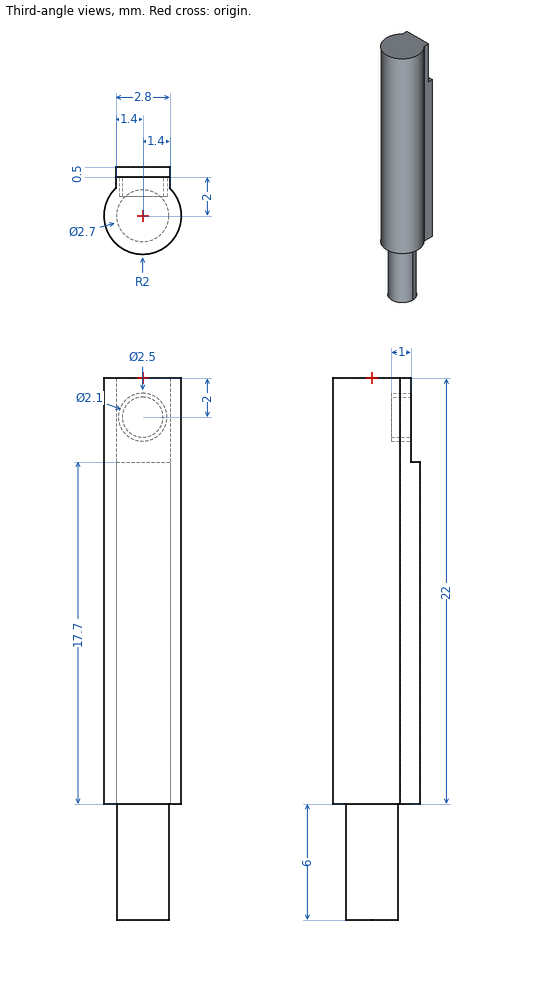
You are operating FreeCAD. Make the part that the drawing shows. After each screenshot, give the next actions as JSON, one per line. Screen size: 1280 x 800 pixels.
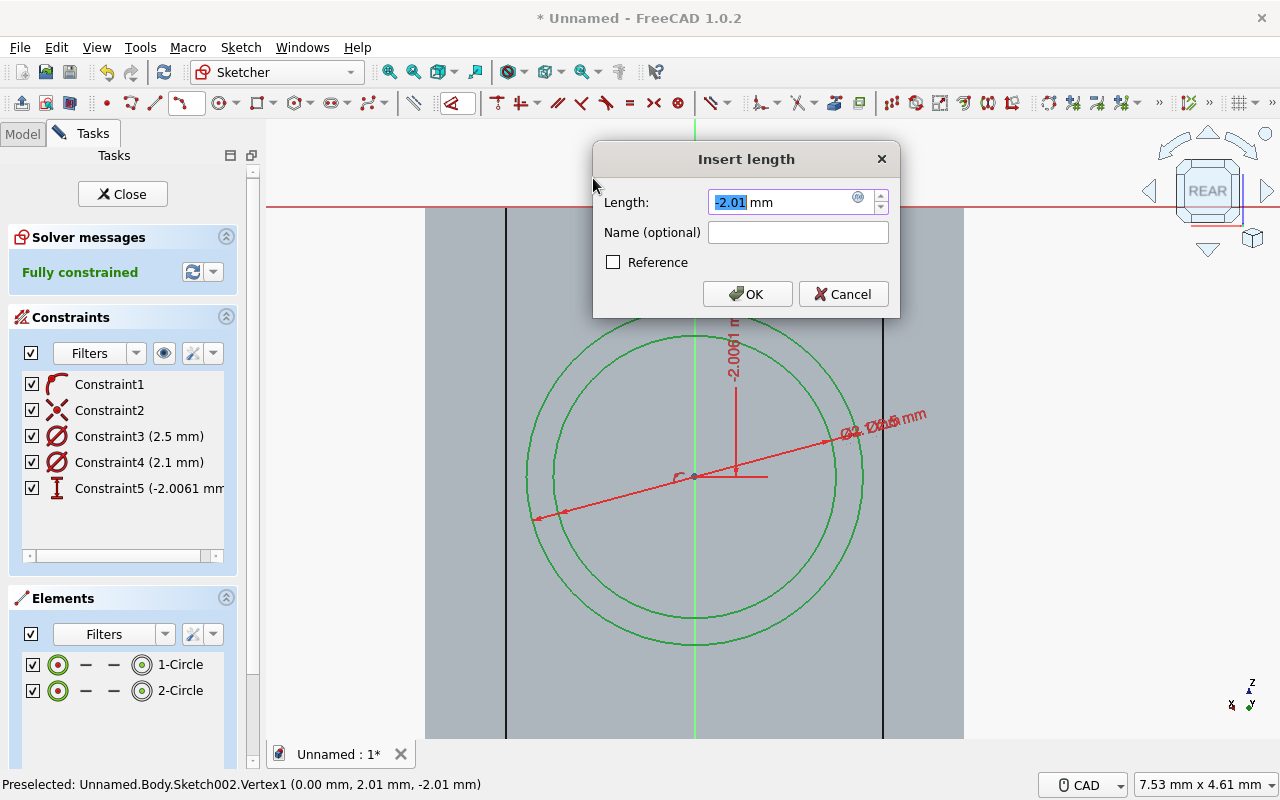
{"action": "type", "text": "-2"}
{"action": "key", "text": "Return"}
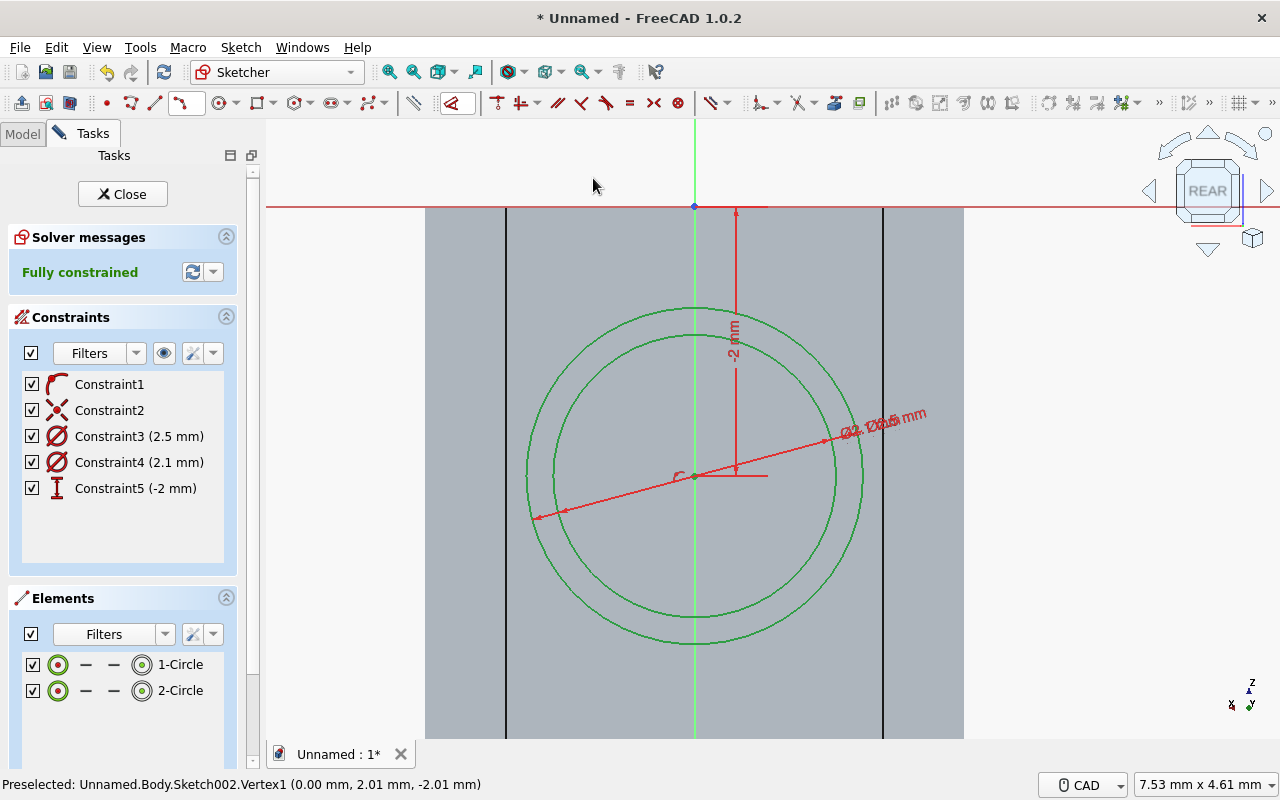
{"action": "left_click", "coordinate": [123, 194]}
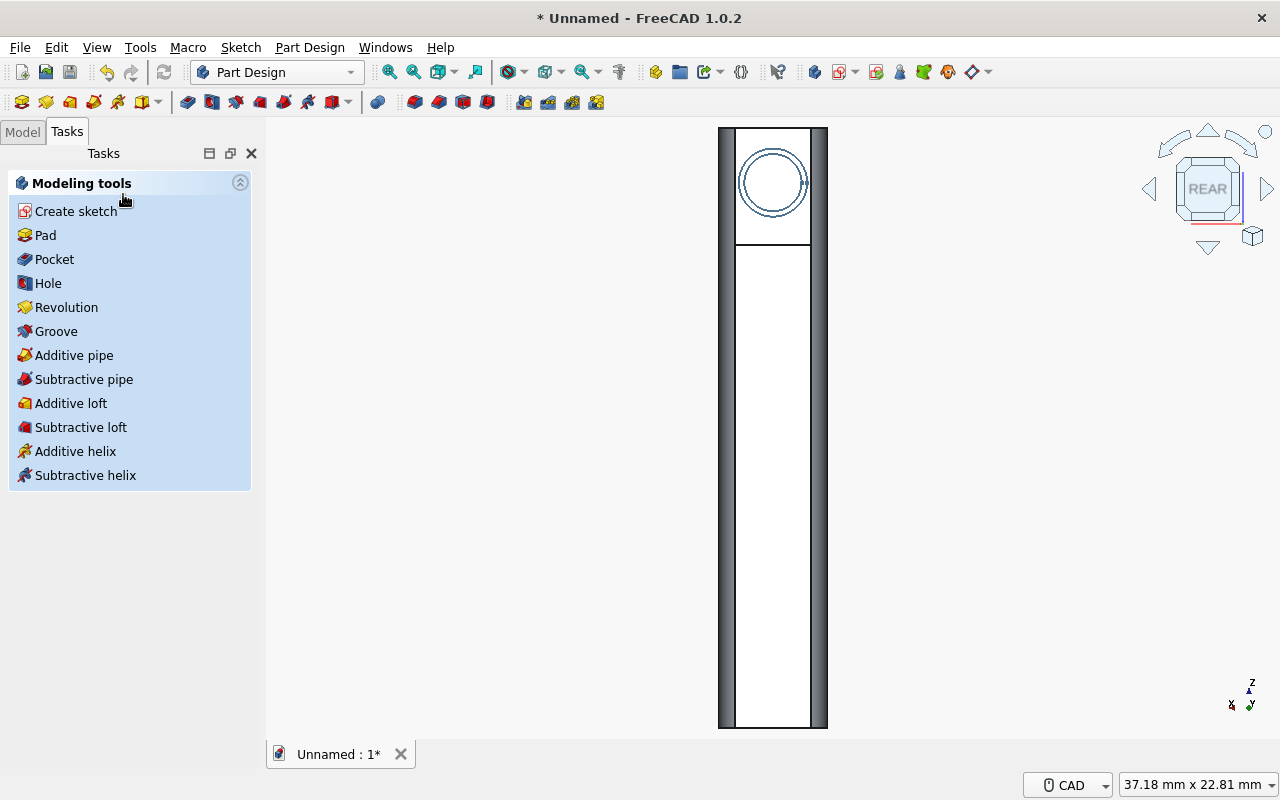
{"action": "left_click", "coordinate": [188, 102]}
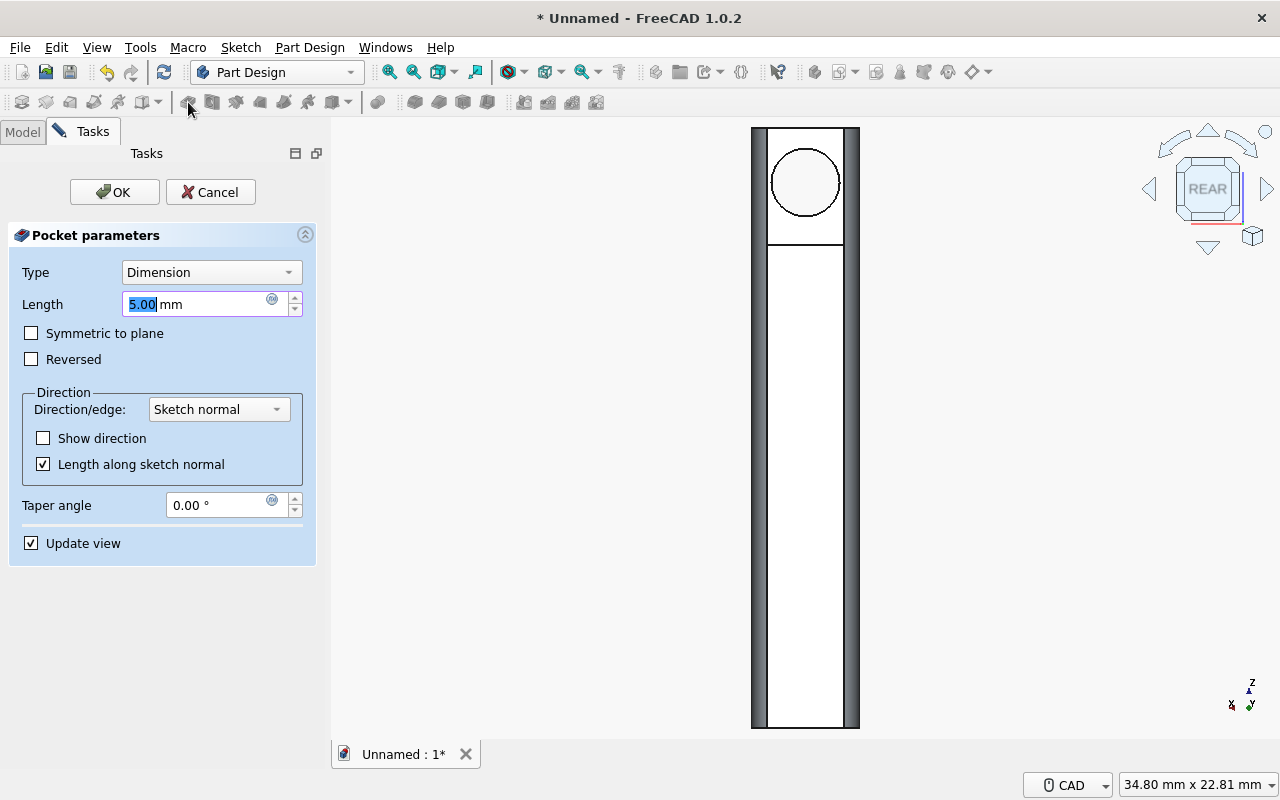
{"action": "type", "text": "1"}
{"action": "key", "text": "Tab"}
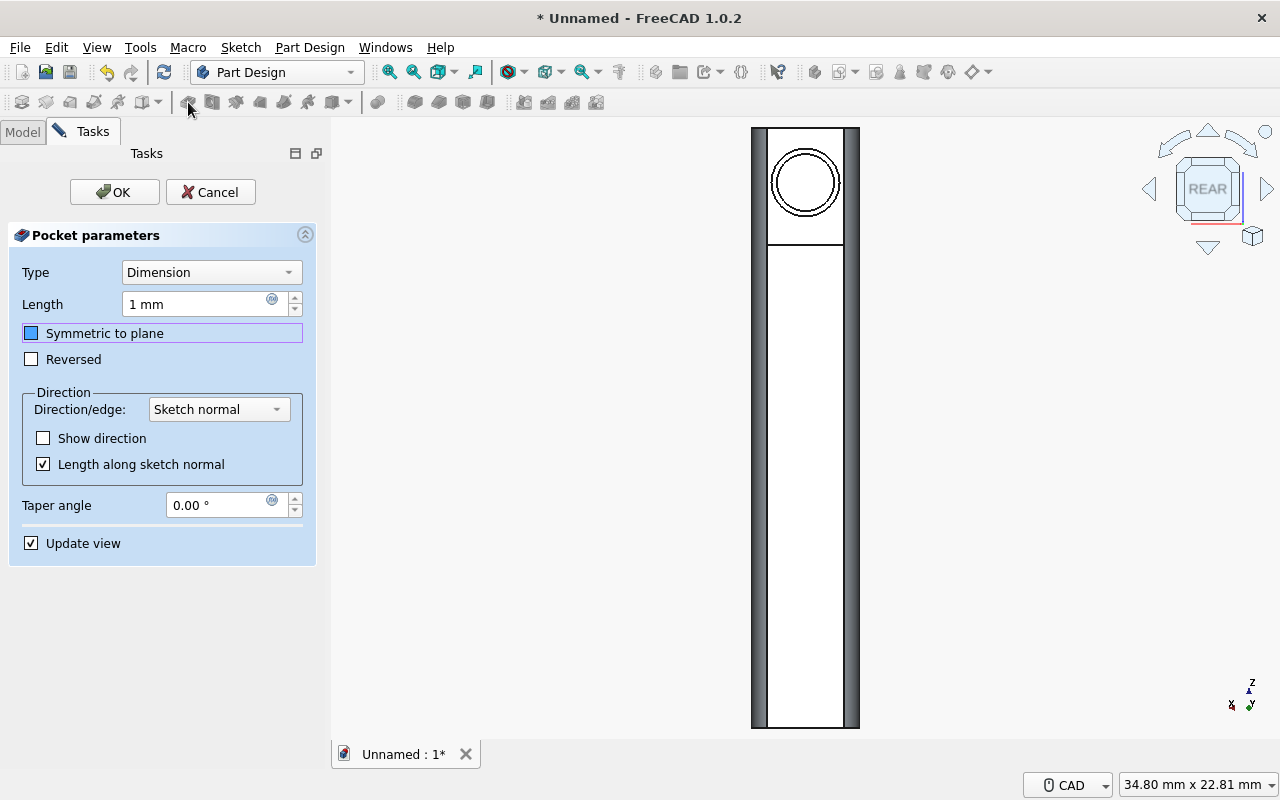
{"action": "left_click", "coordinate": [115, 192]}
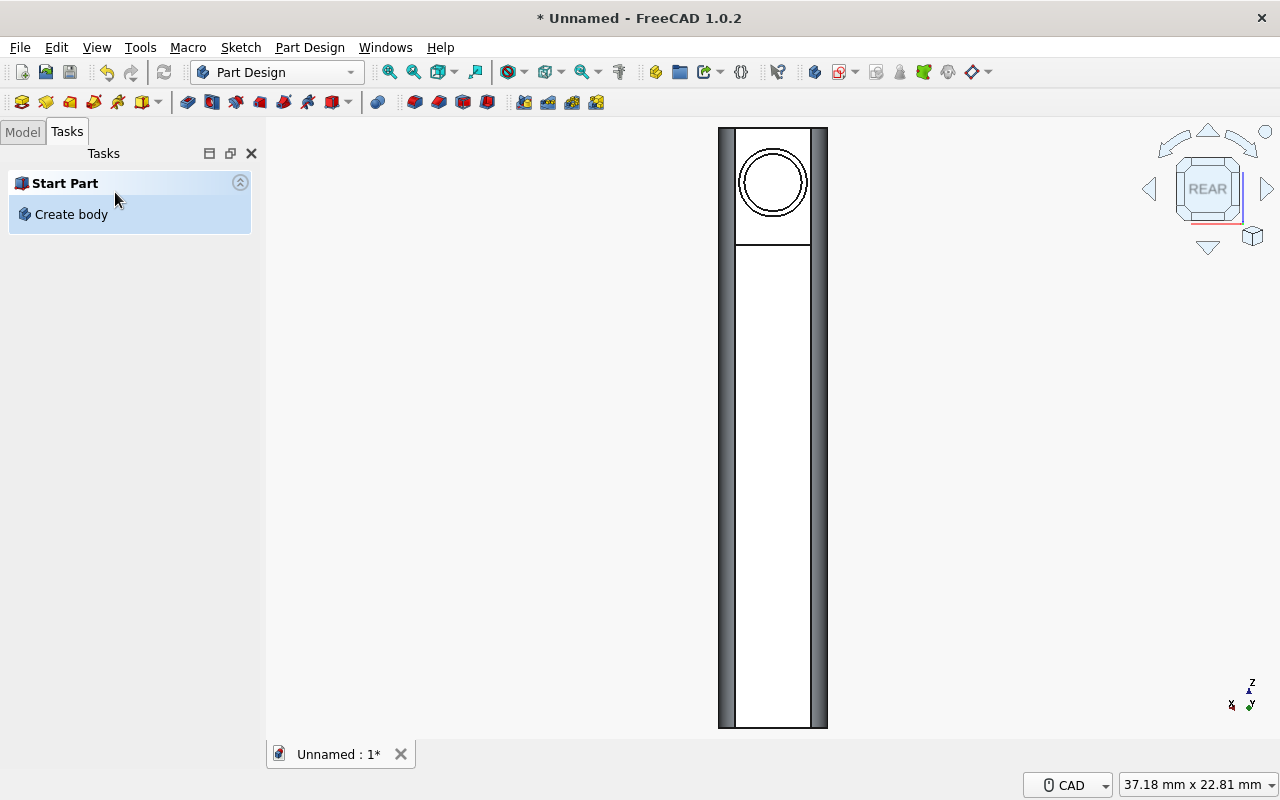
{"action": "key", "text": "5"}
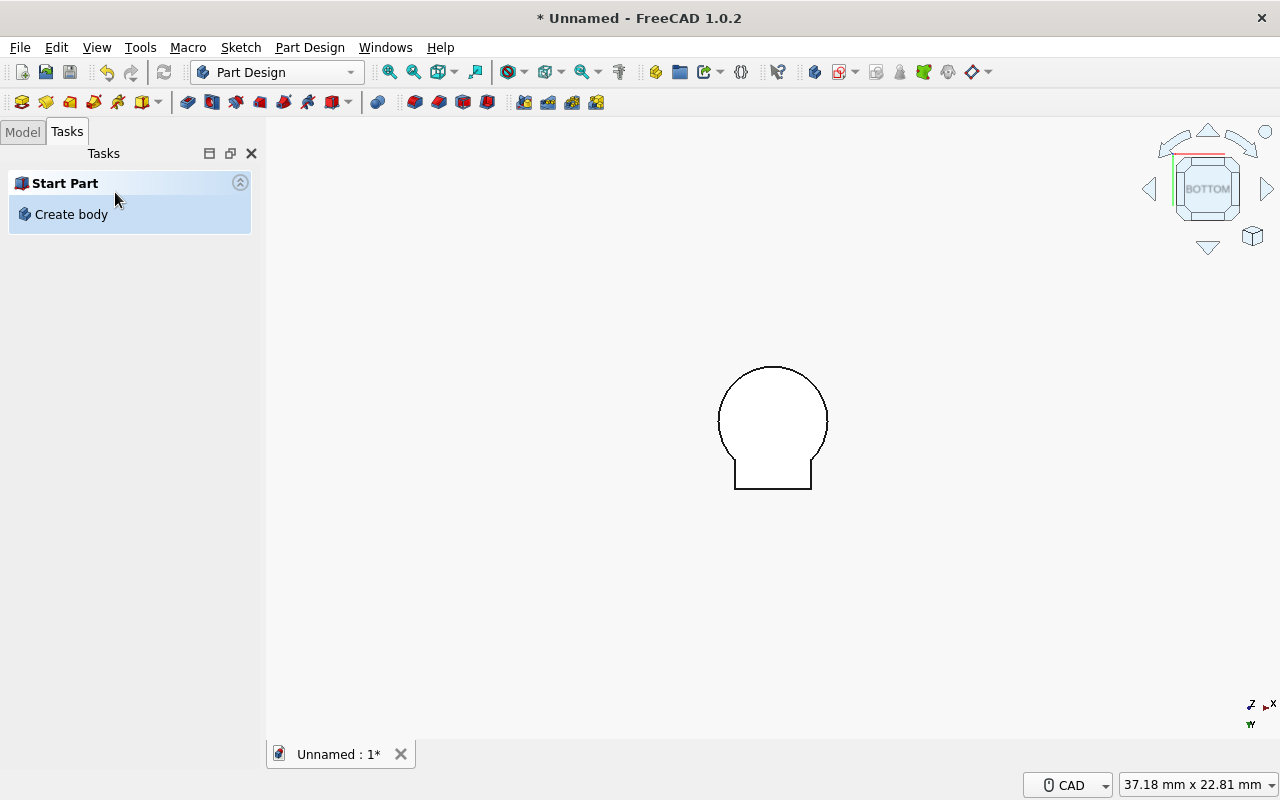
{"action": "left_click", "coordinate": [390, 72]}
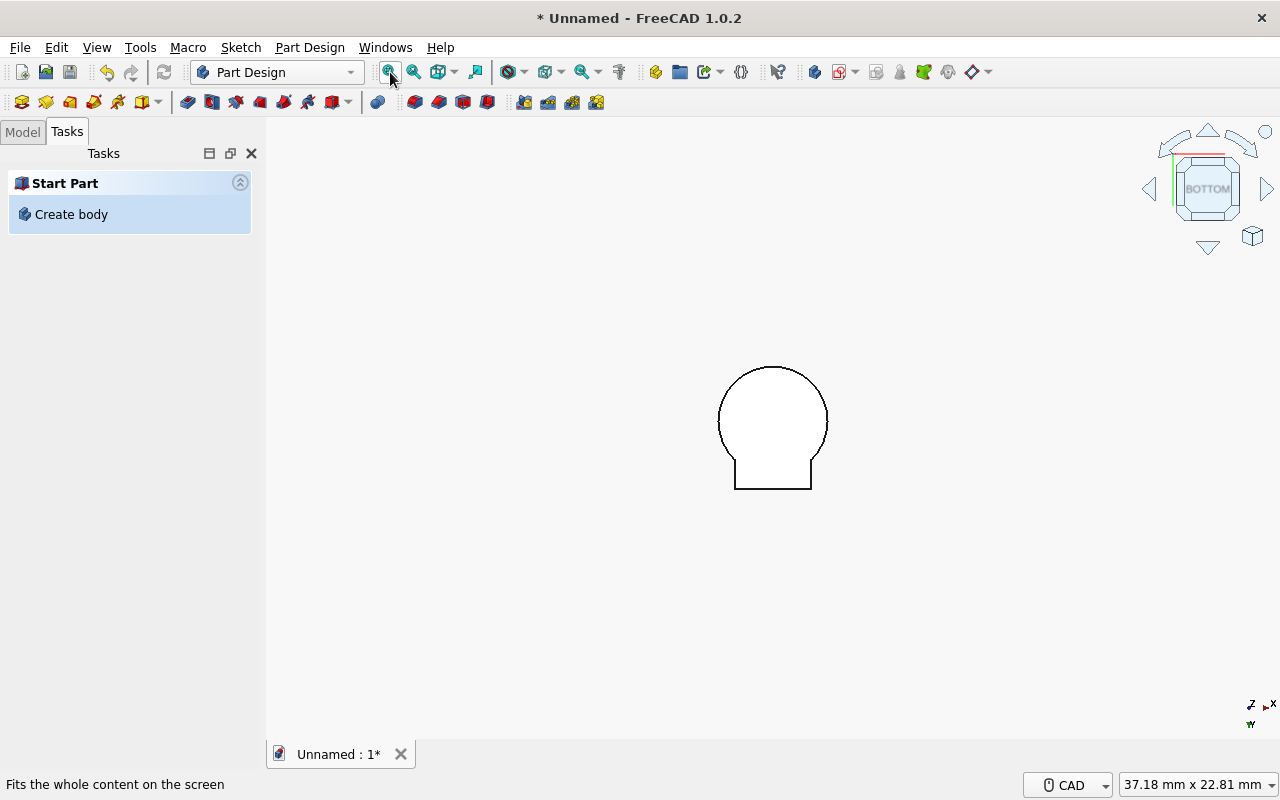
{"action": "left_click", "coordinate": [773, 427]}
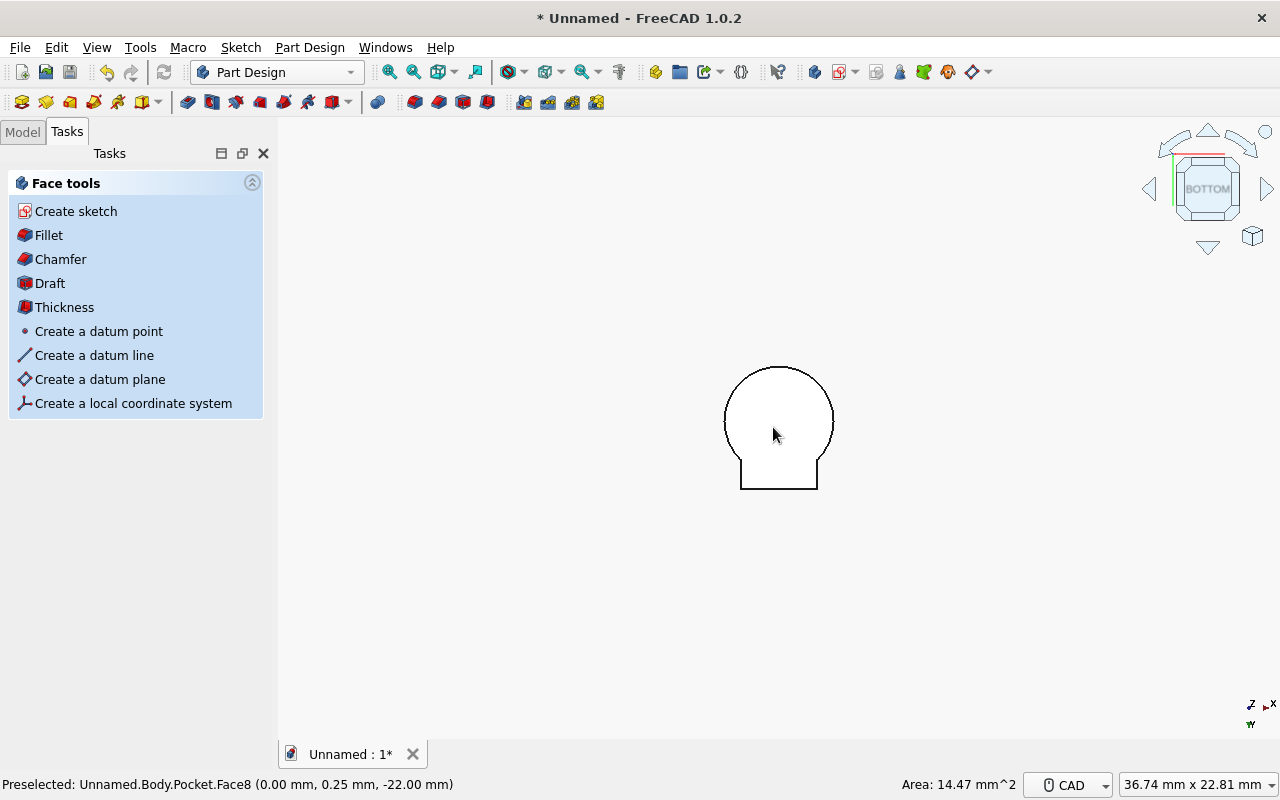
{"action": "left_click", "coordinate": [840, 72]}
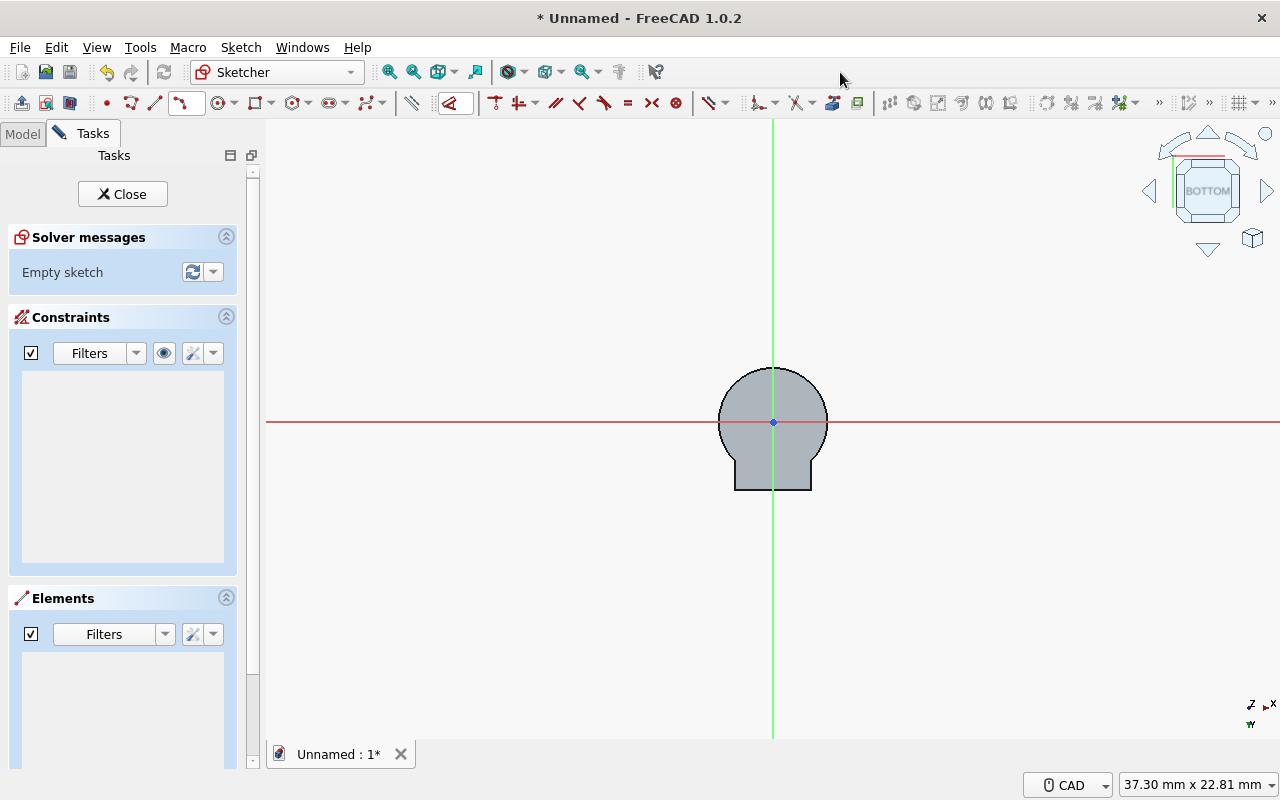
{"action": "scroll", "coordinate": [790, 420], "scroll_direction": "up", "scroll_amount": 8}